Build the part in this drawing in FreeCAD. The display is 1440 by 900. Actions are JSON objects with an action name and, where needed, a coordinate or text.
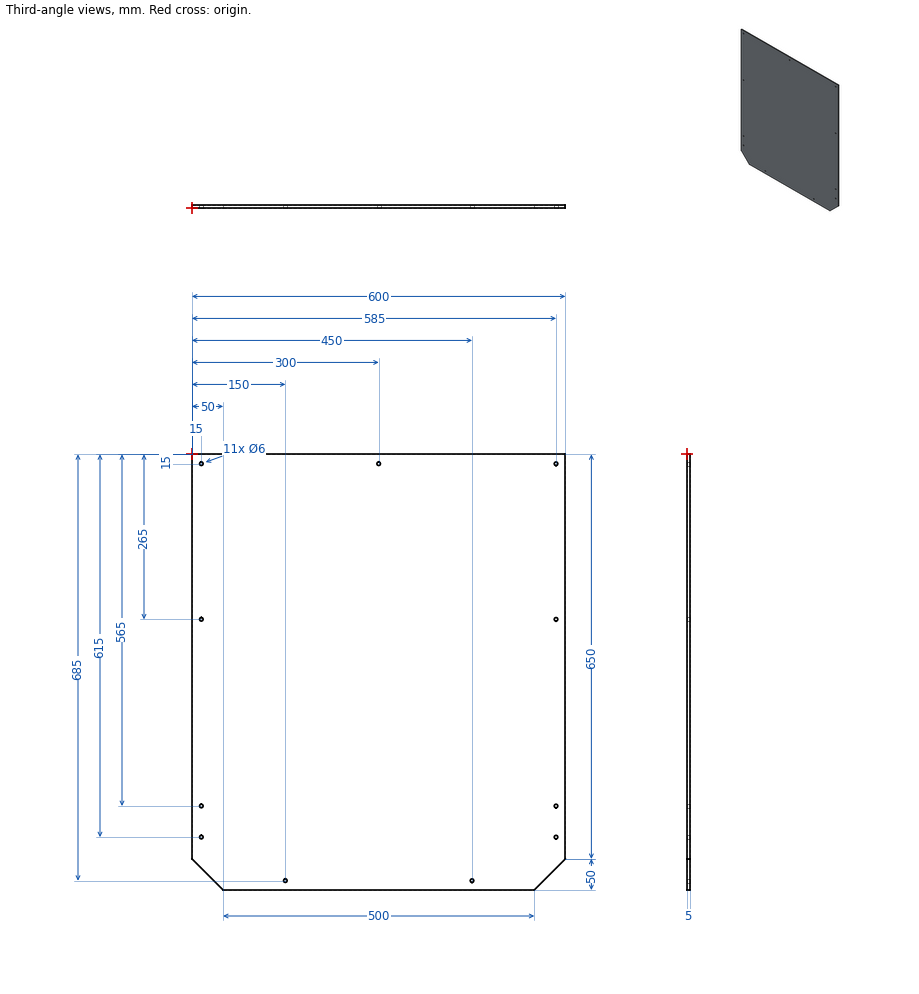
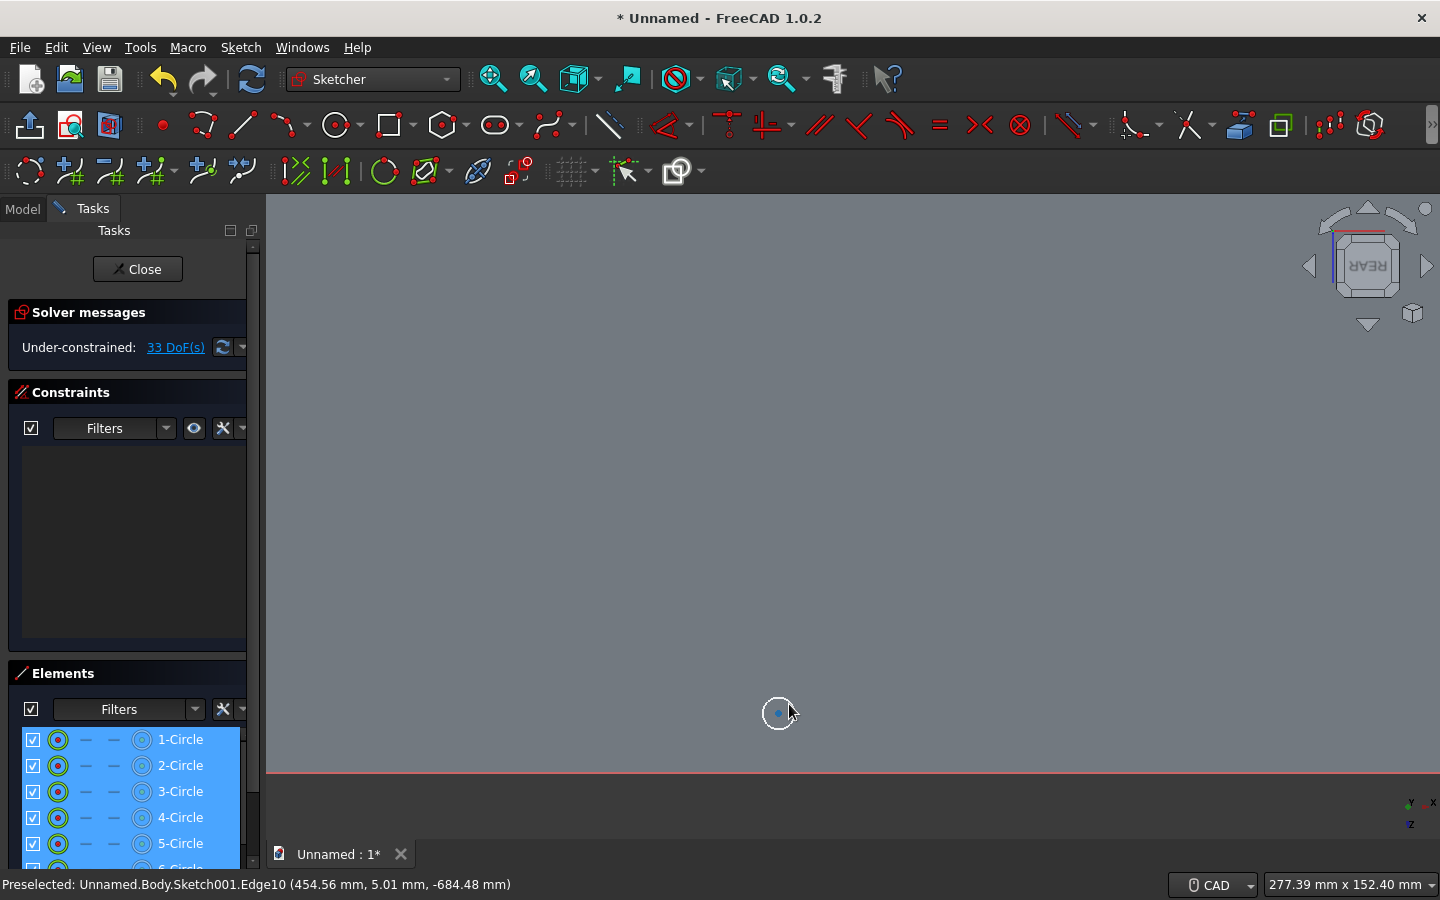
{"action": "left_click", "coordinate": [790, 702]}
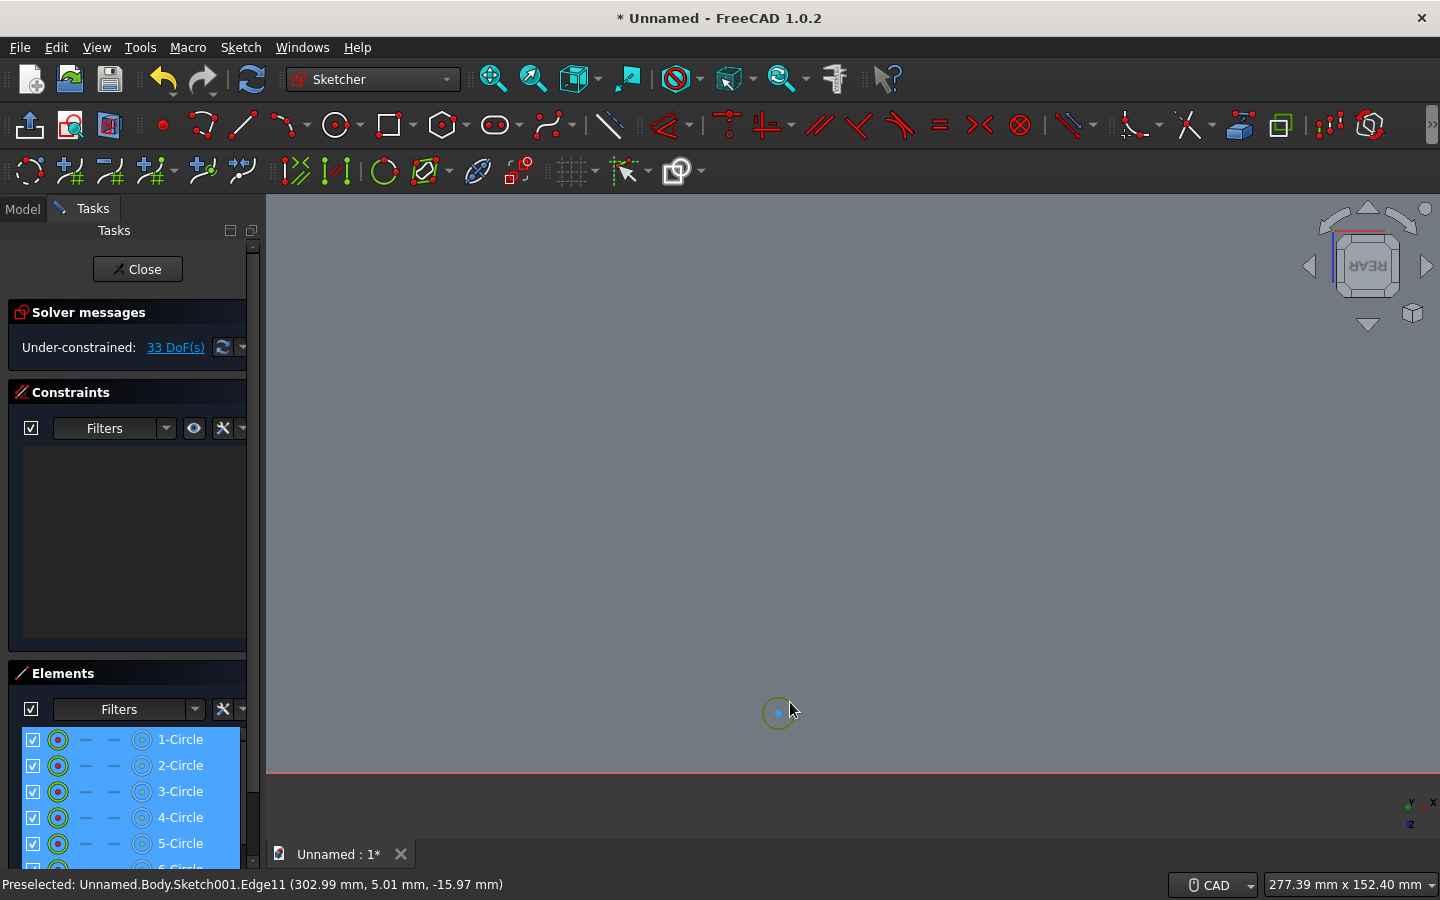
{"action": "left_click", "coordinate": [940, 126]}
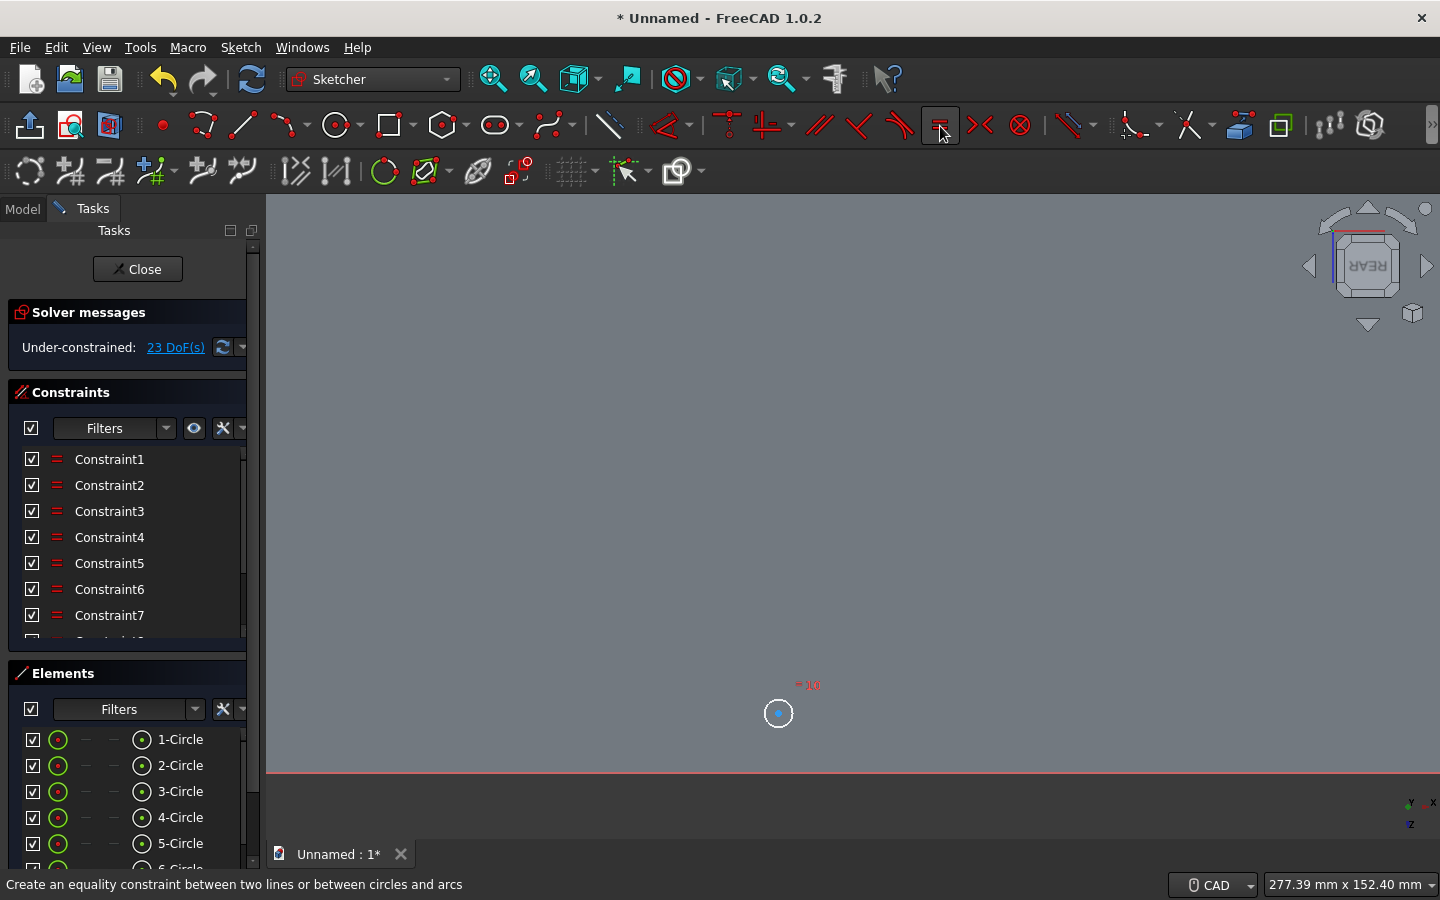
{"action": "scroll", "coordinate": [789, 704], "scroll_direction": "down", "scroll_amount": 10}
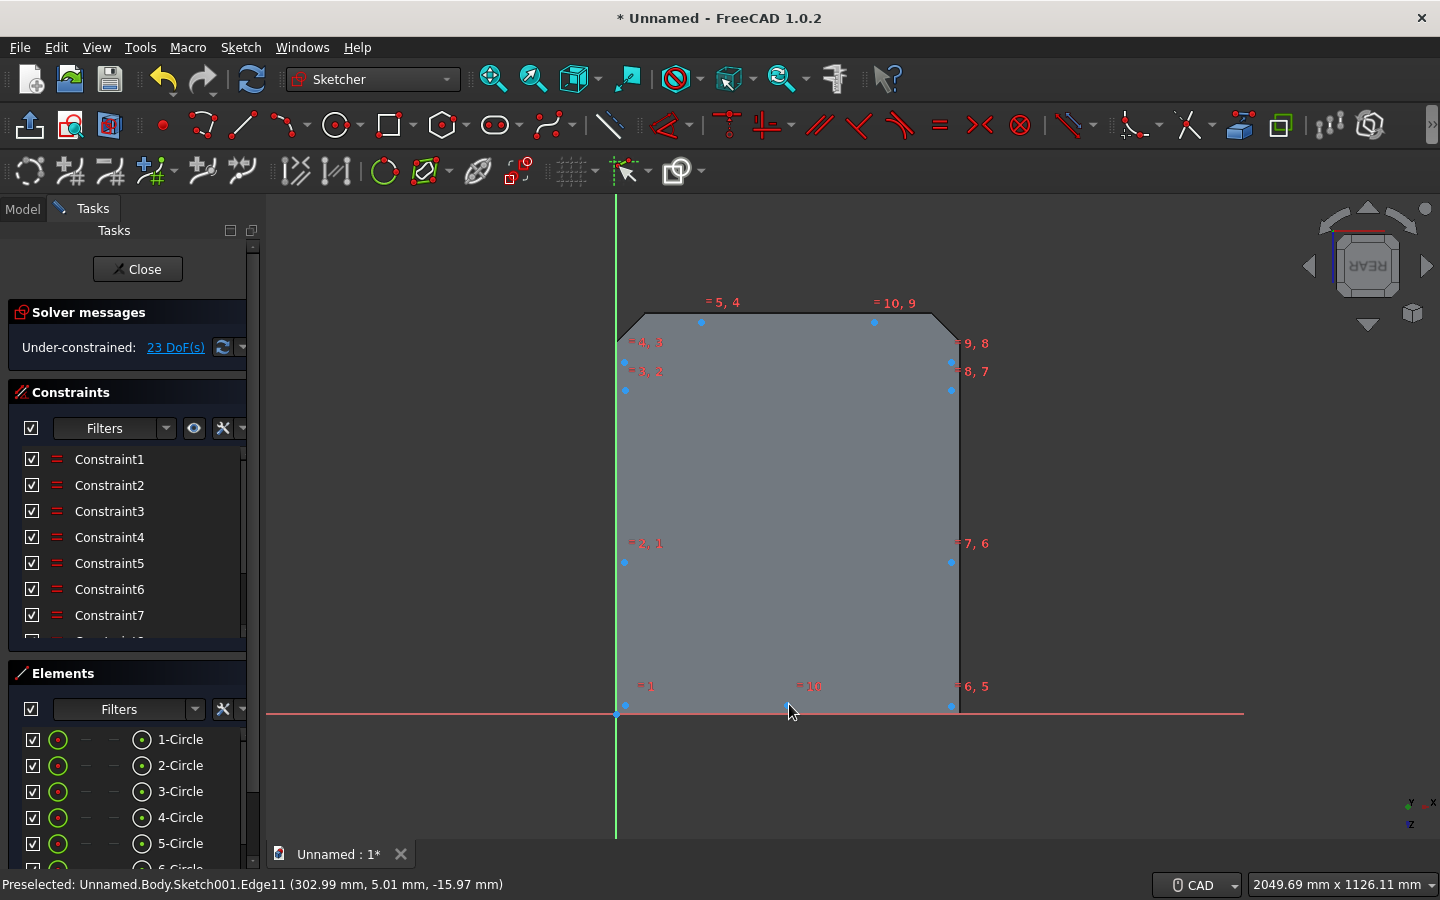
{"action": "left_click", "coordinate": [625, 706]}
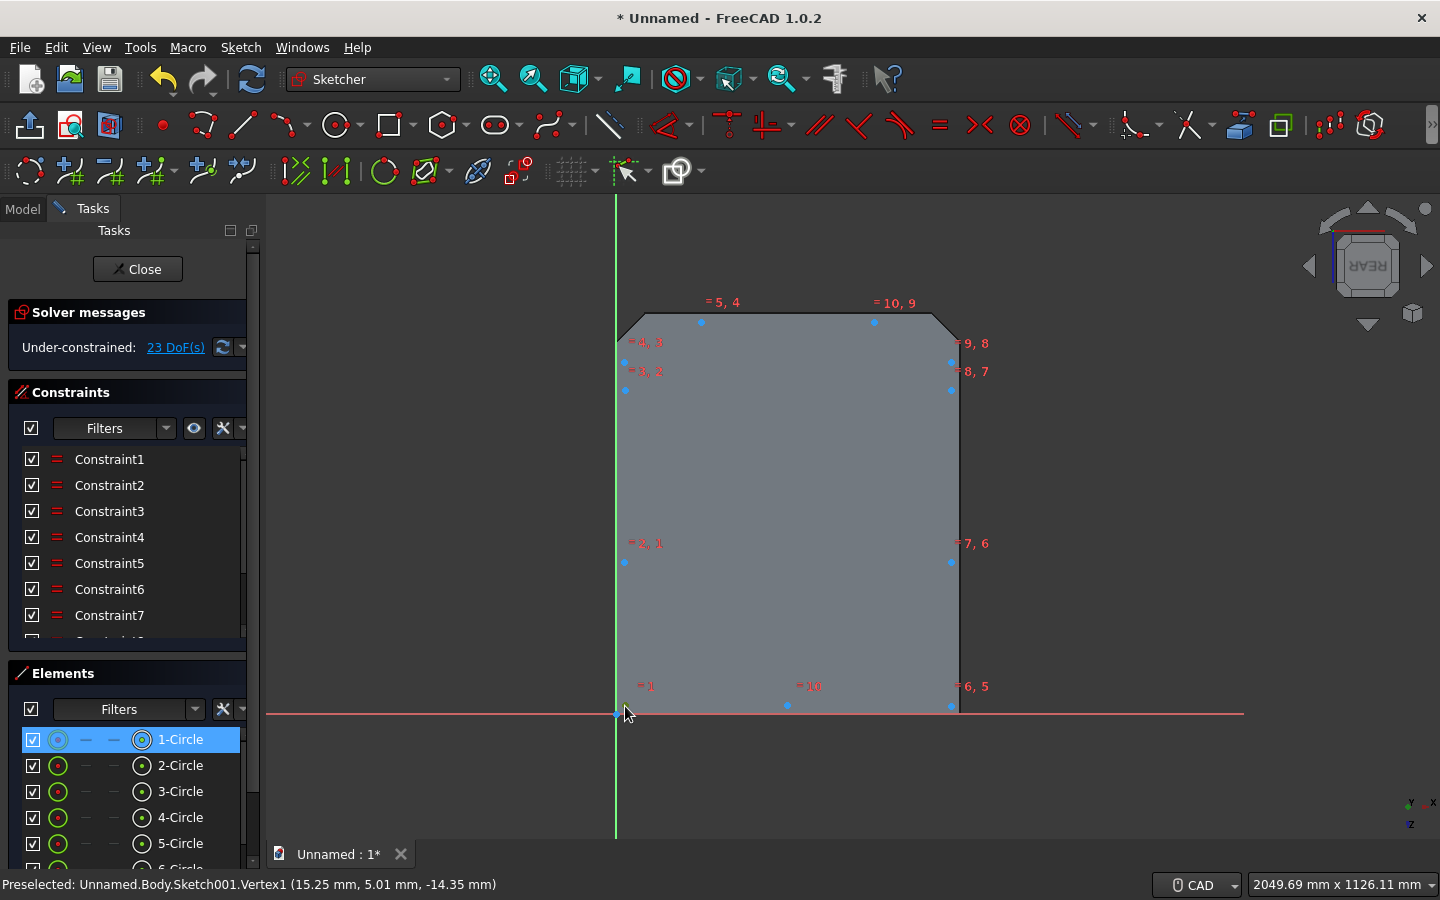
{"action": "left_click", "coordinate": [625, 563]}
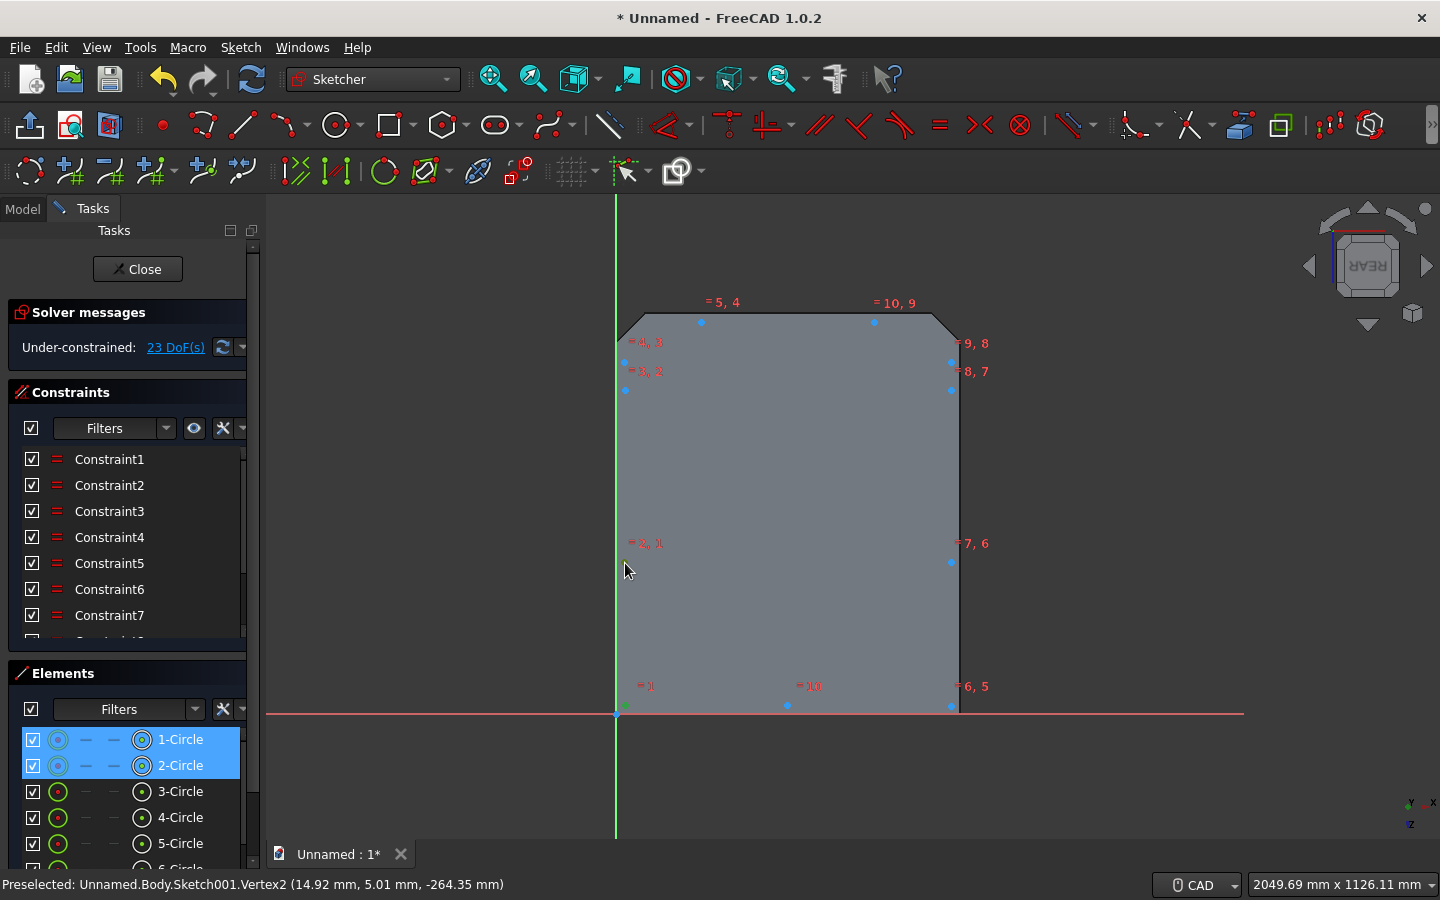
{"action": "key", "text": "v"}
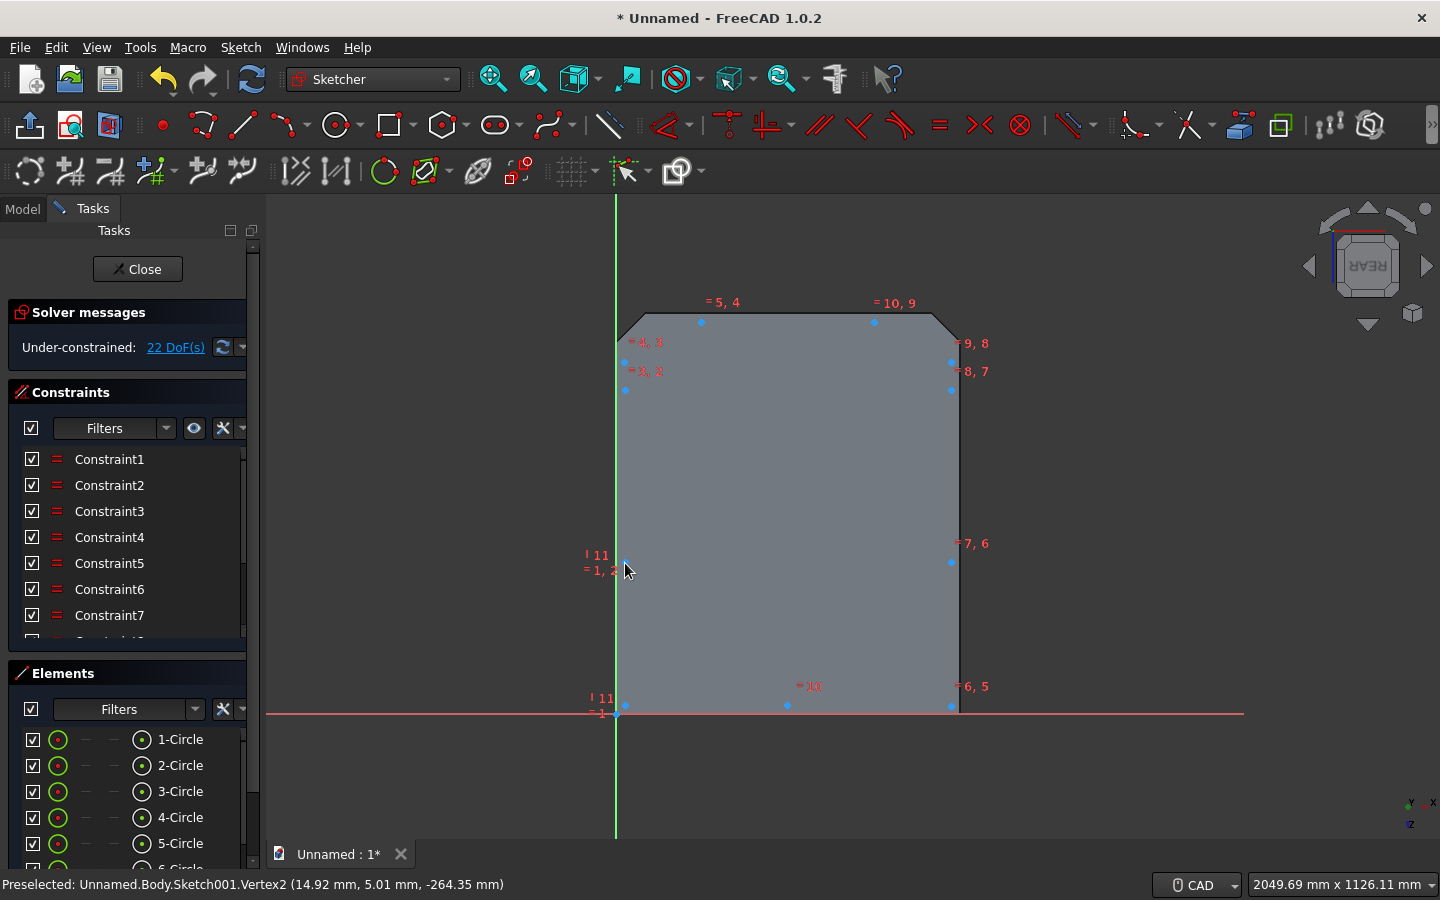
{"action": "left_click", "coordinate": [625, 563]}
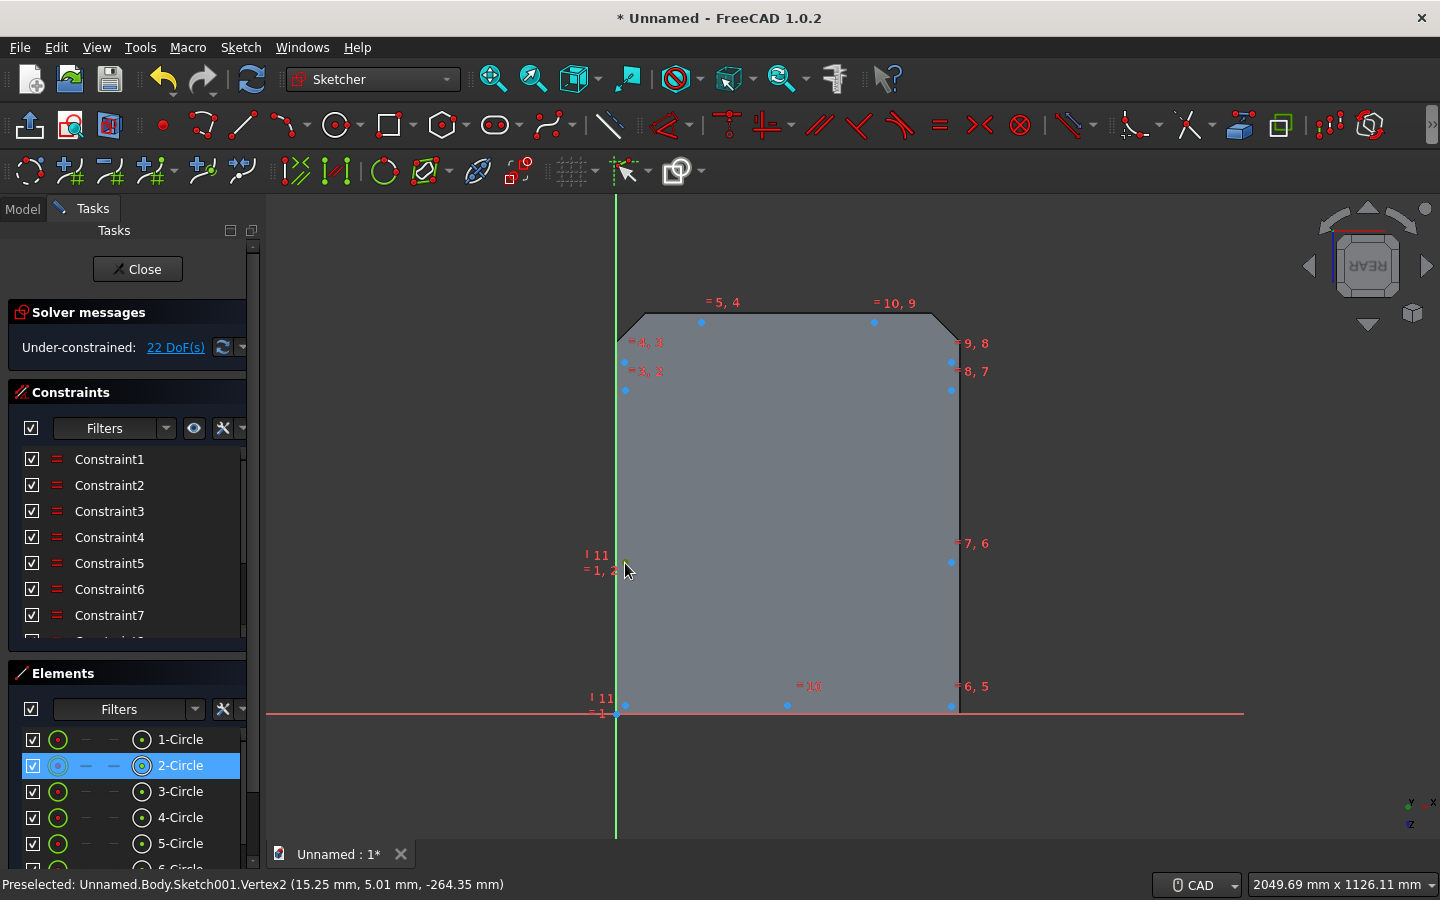
{"action": "left_click", "coordinate": [625, 391]}